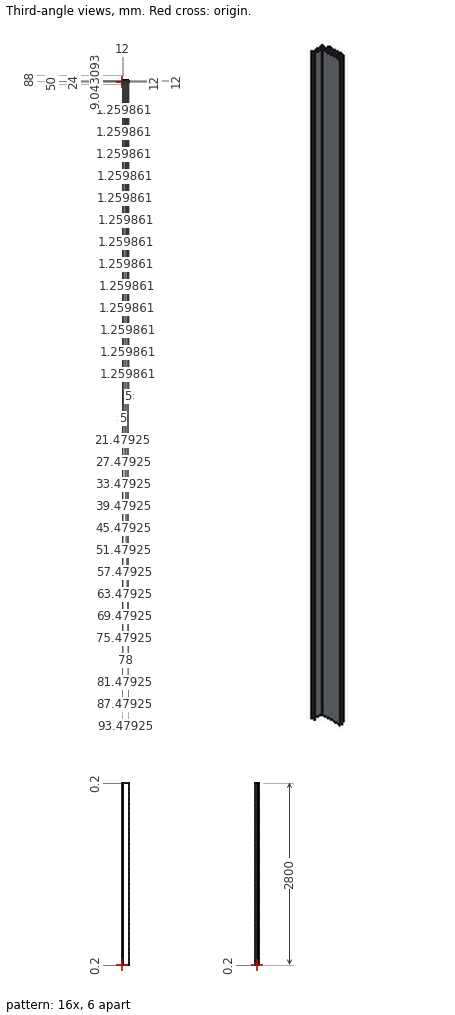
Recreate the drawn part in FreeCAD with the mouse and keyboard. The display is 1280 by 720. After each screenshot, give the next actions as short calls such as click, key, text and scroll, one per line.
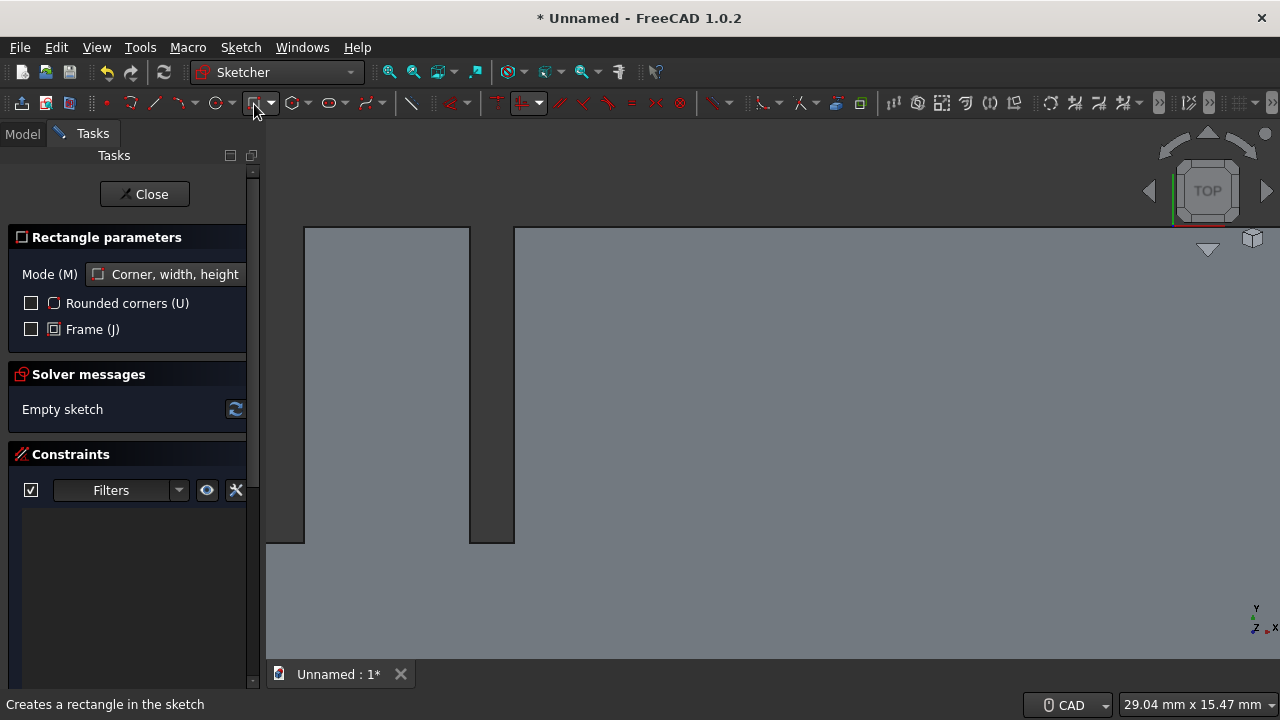
click(679, 227)
move(723, 543)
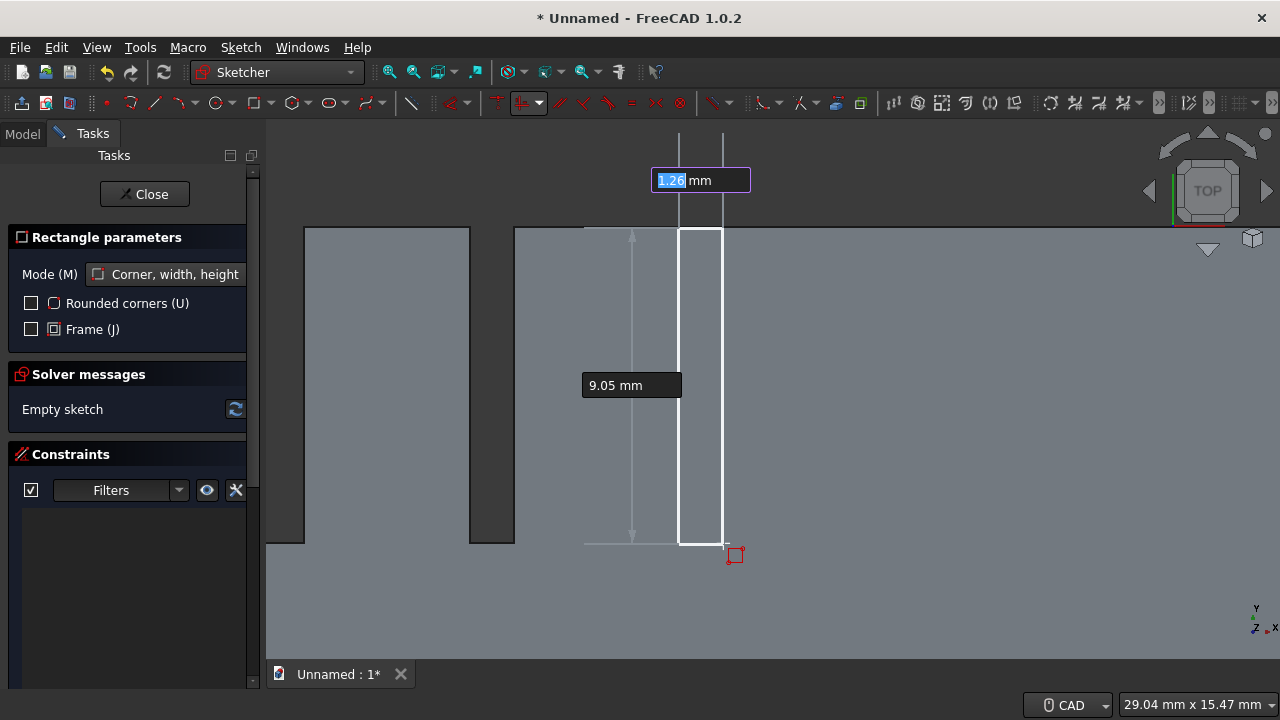
text(1.259861)
key(Tab)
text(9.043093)
key(Return)
key(Escape)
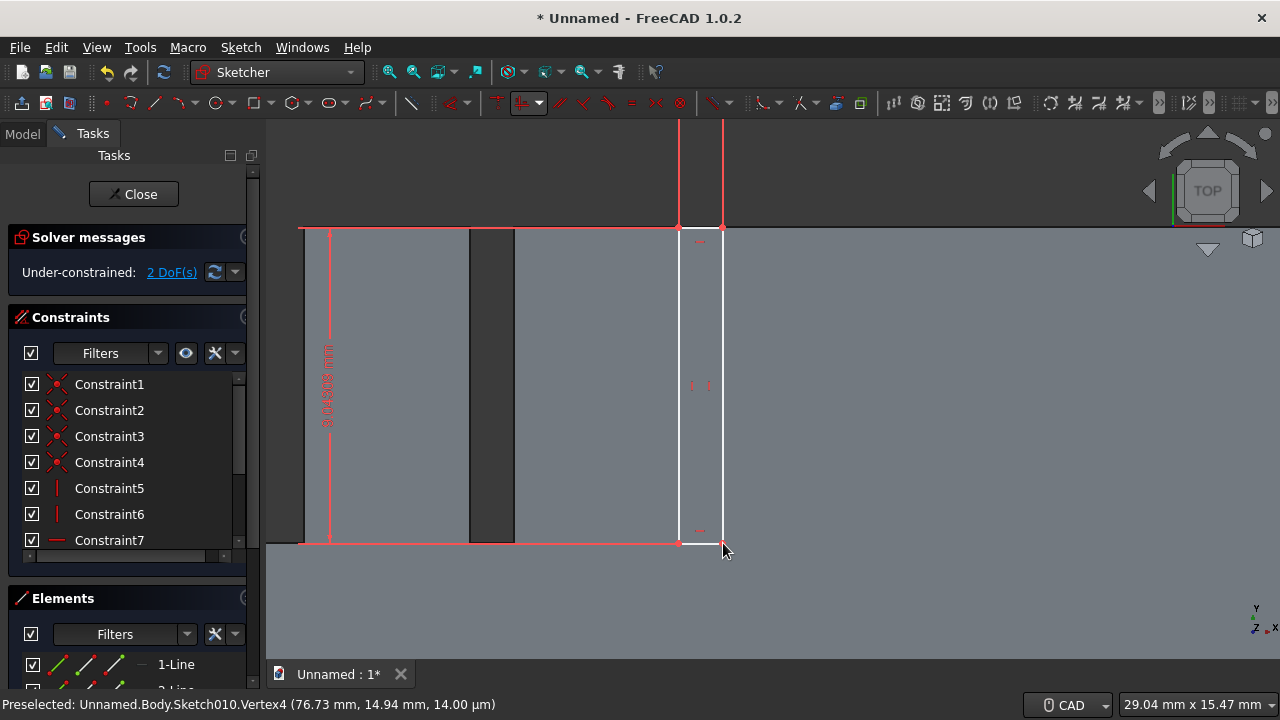
click(450, 104)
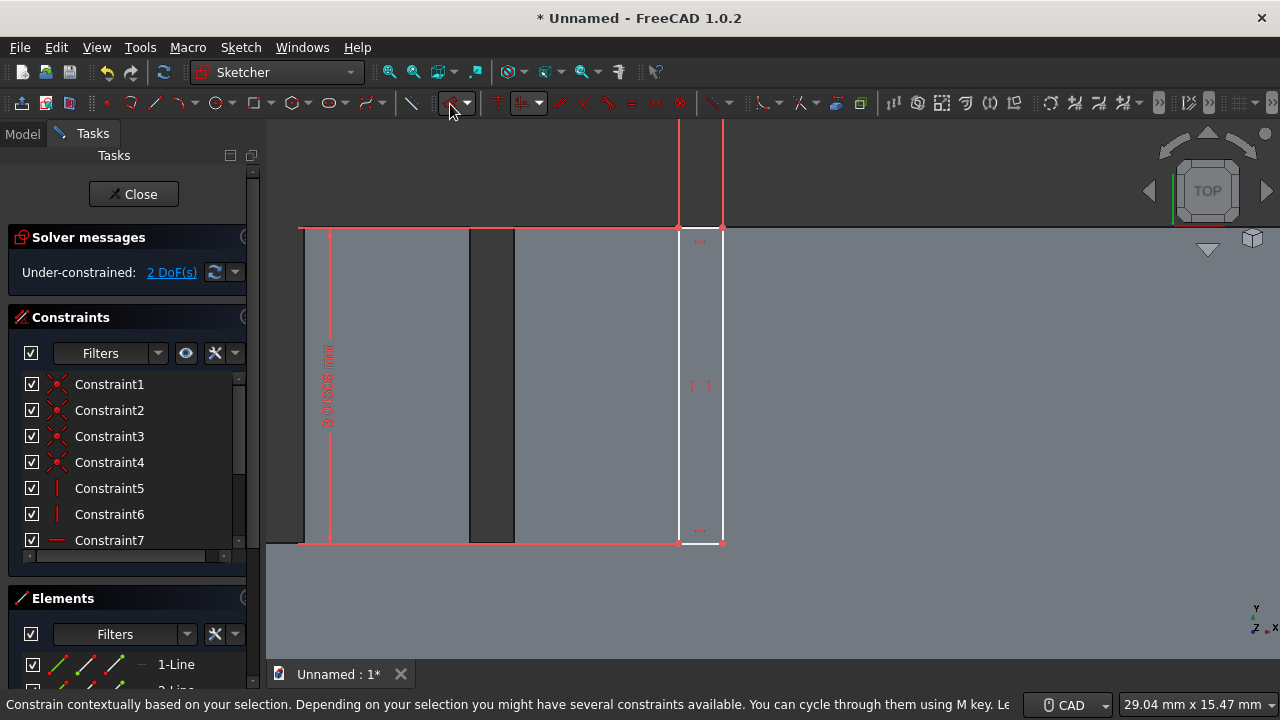
click(679, 228)
click(713, 571)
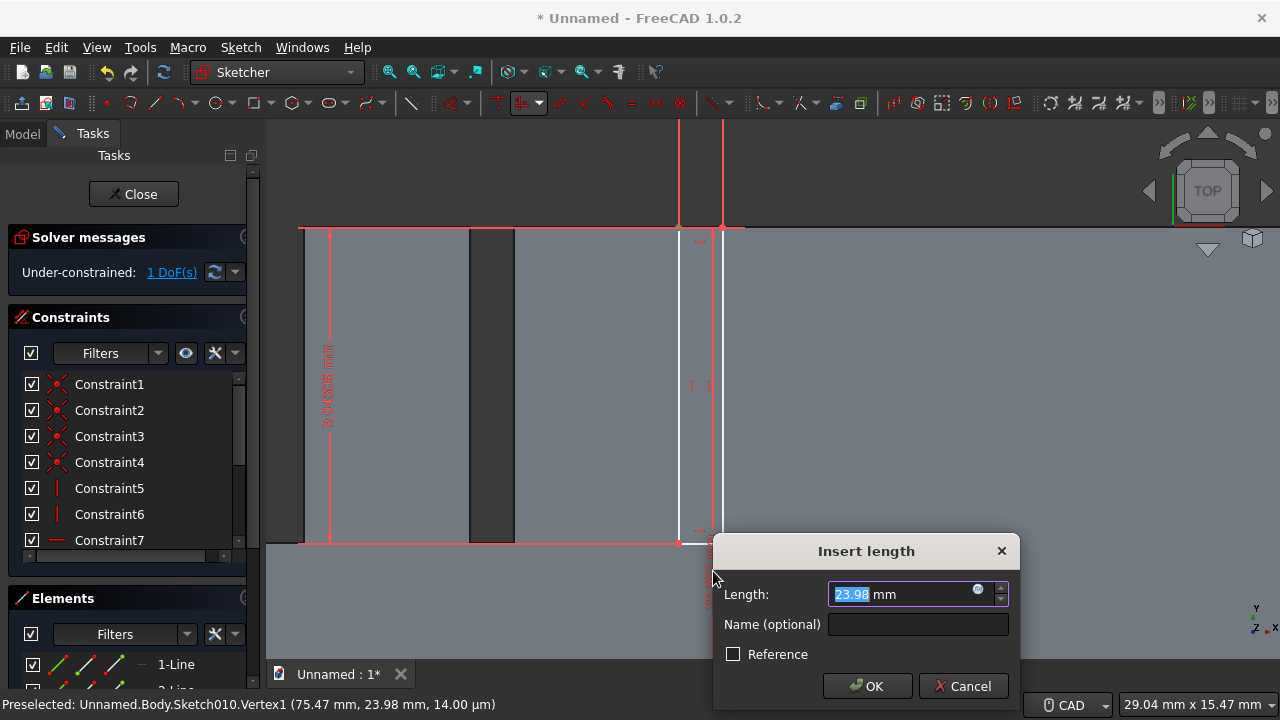
text(24)
key(Return)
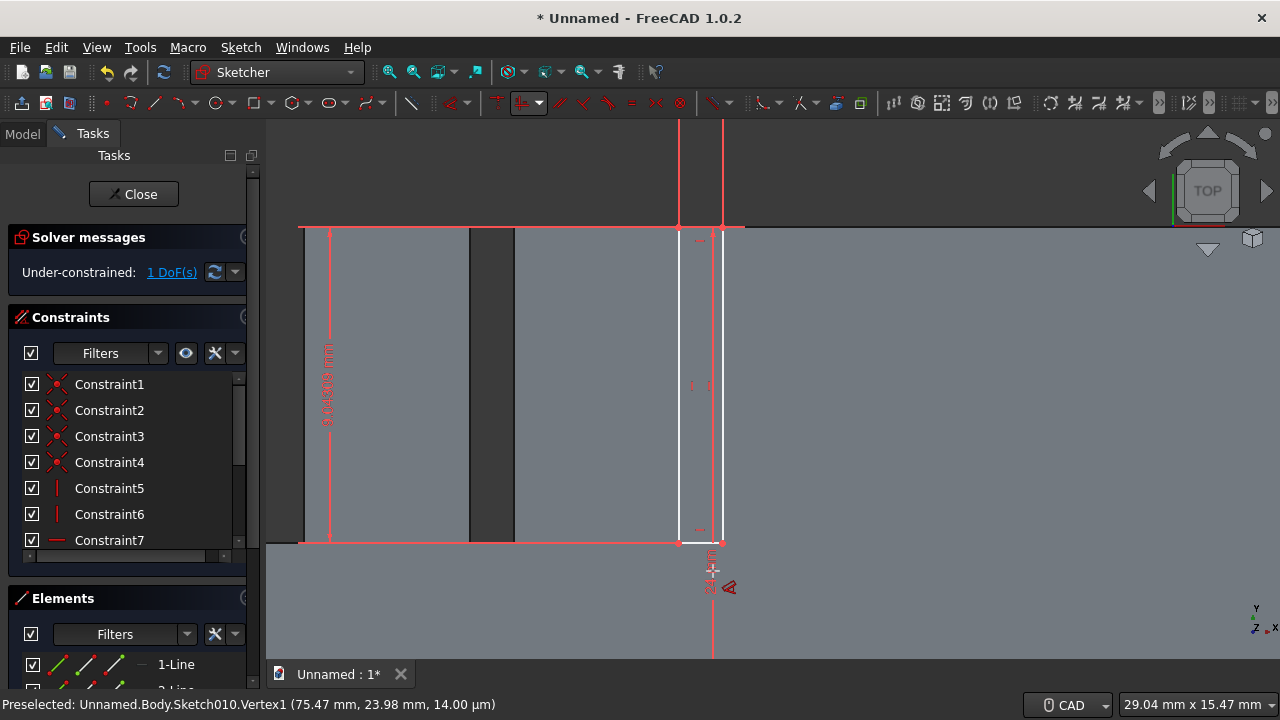
click(679, 227)
click(486, 193)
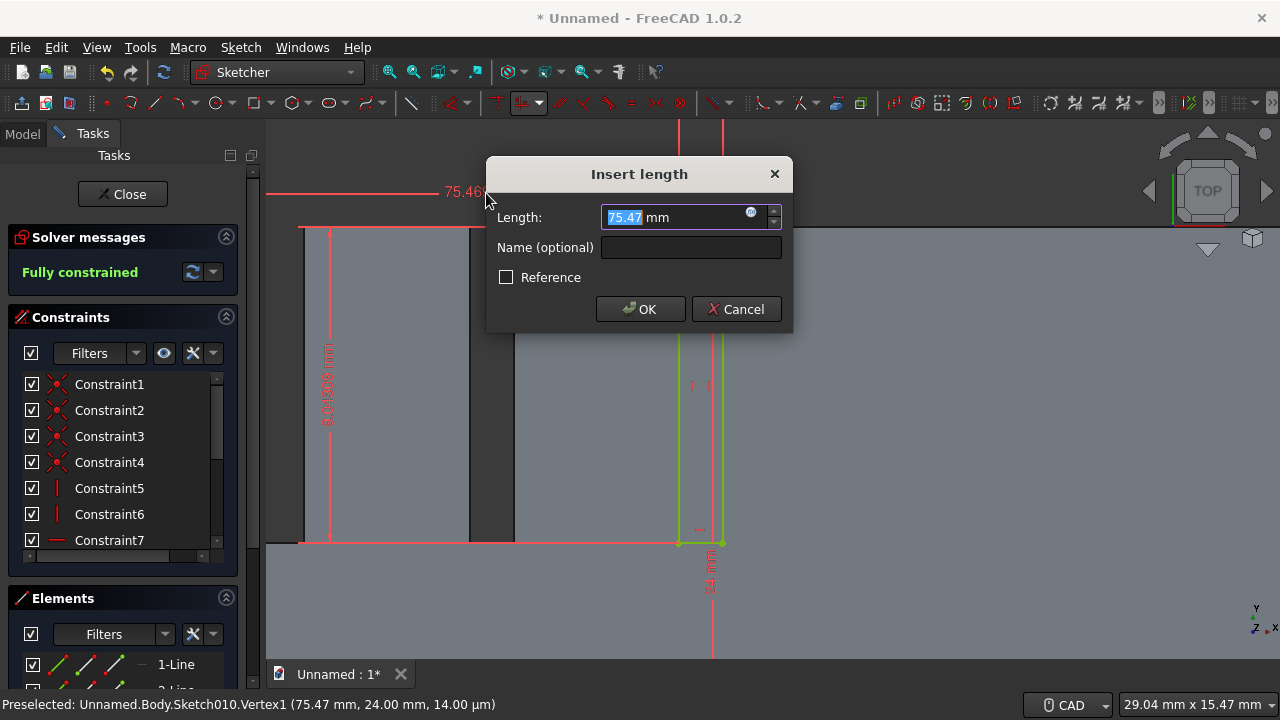
text(75.47925)
key(Return)
key(Escape)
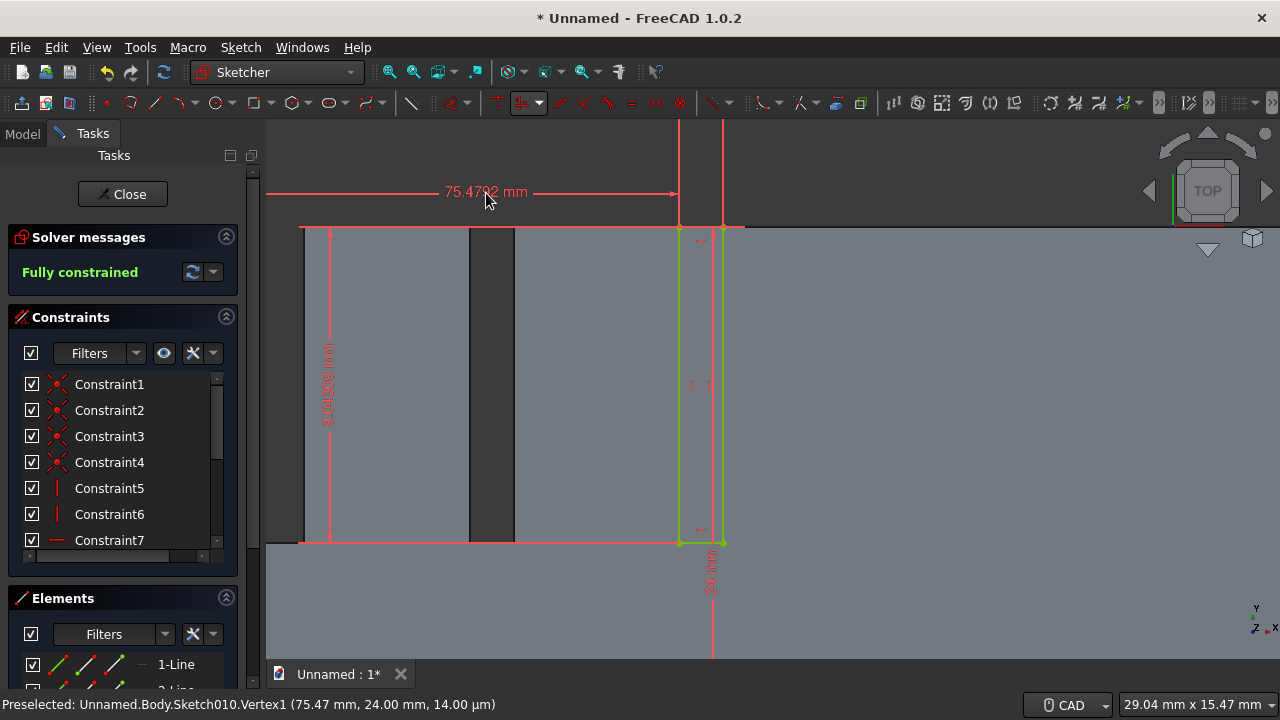
click(123, 194)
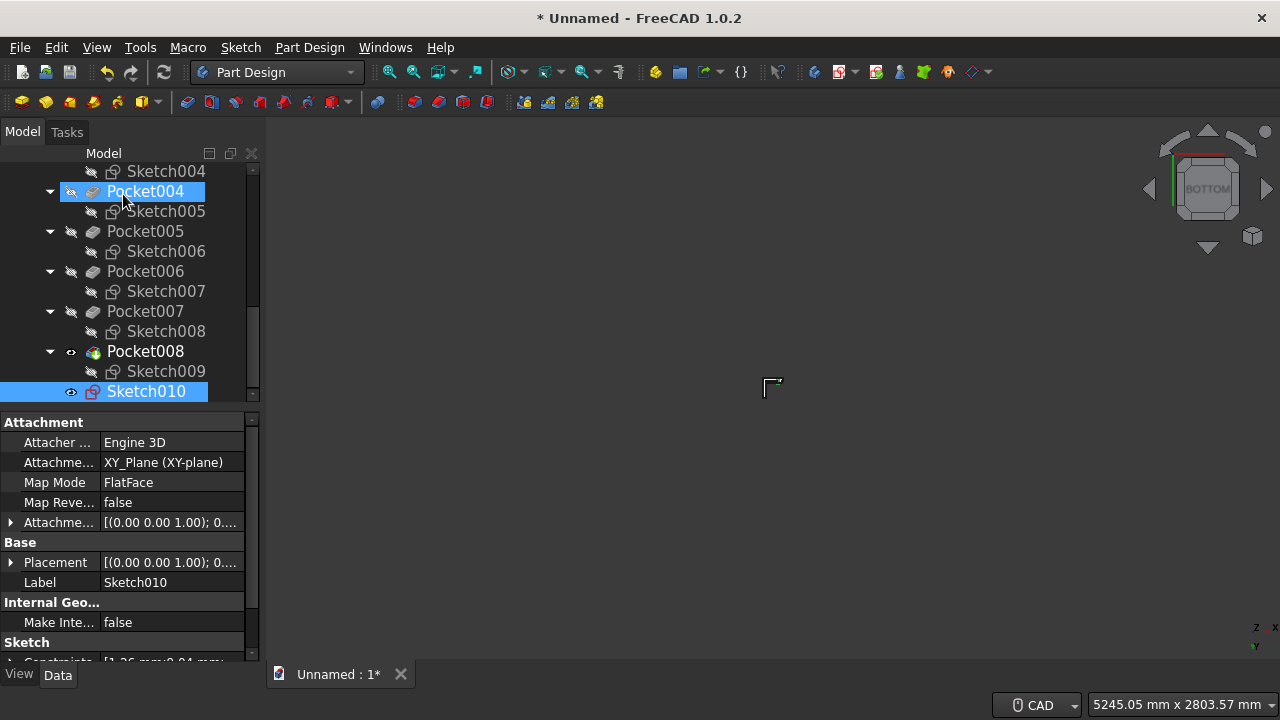
click(188, 102)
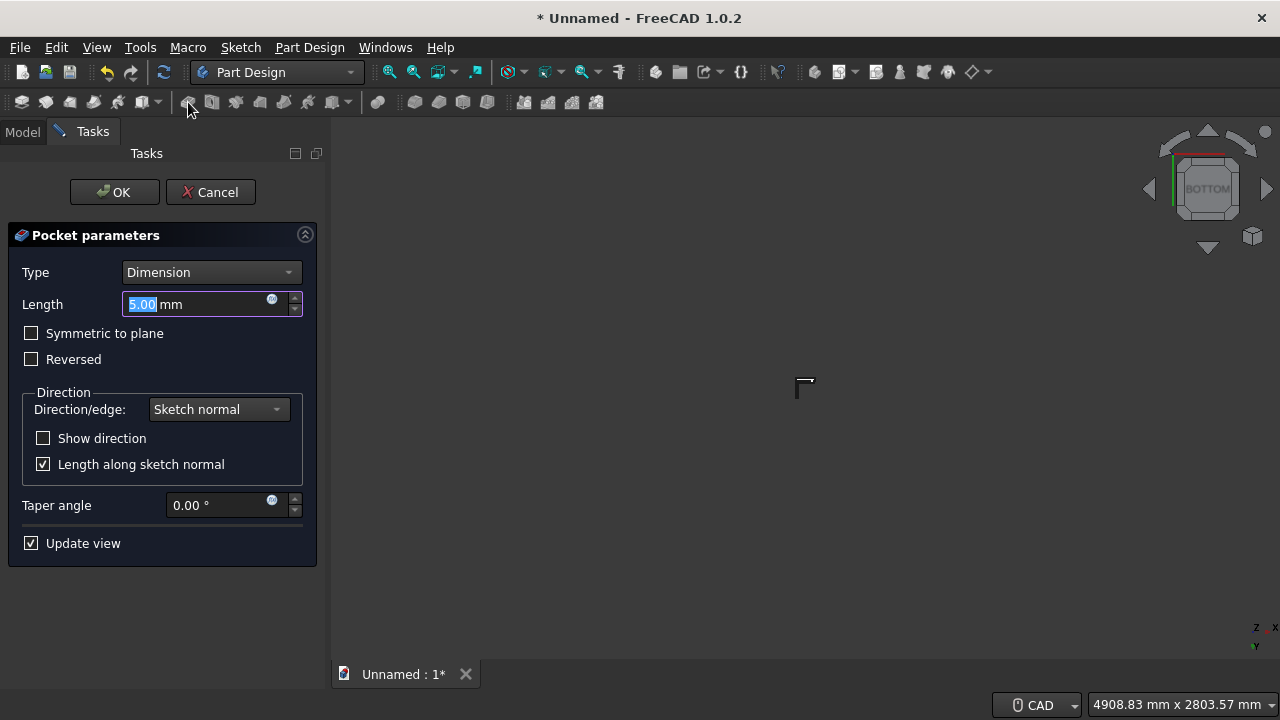
text(0.2)
key(Tab)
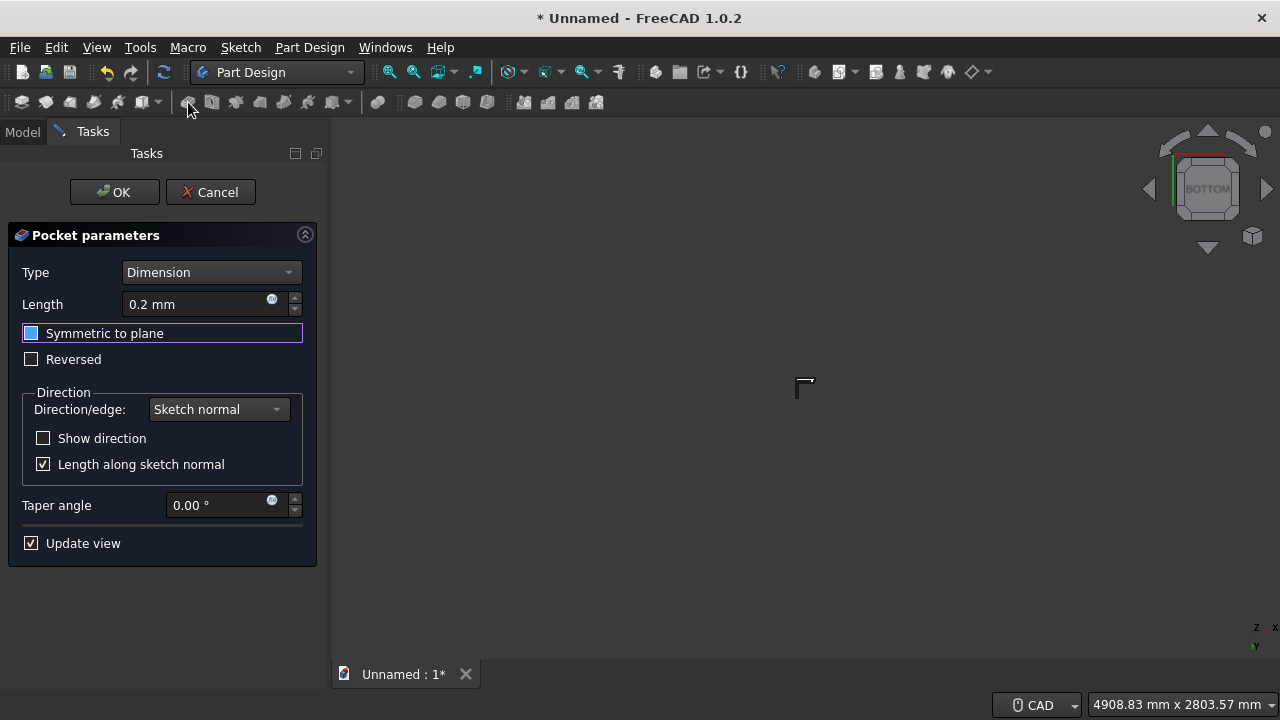
click(30, 359)